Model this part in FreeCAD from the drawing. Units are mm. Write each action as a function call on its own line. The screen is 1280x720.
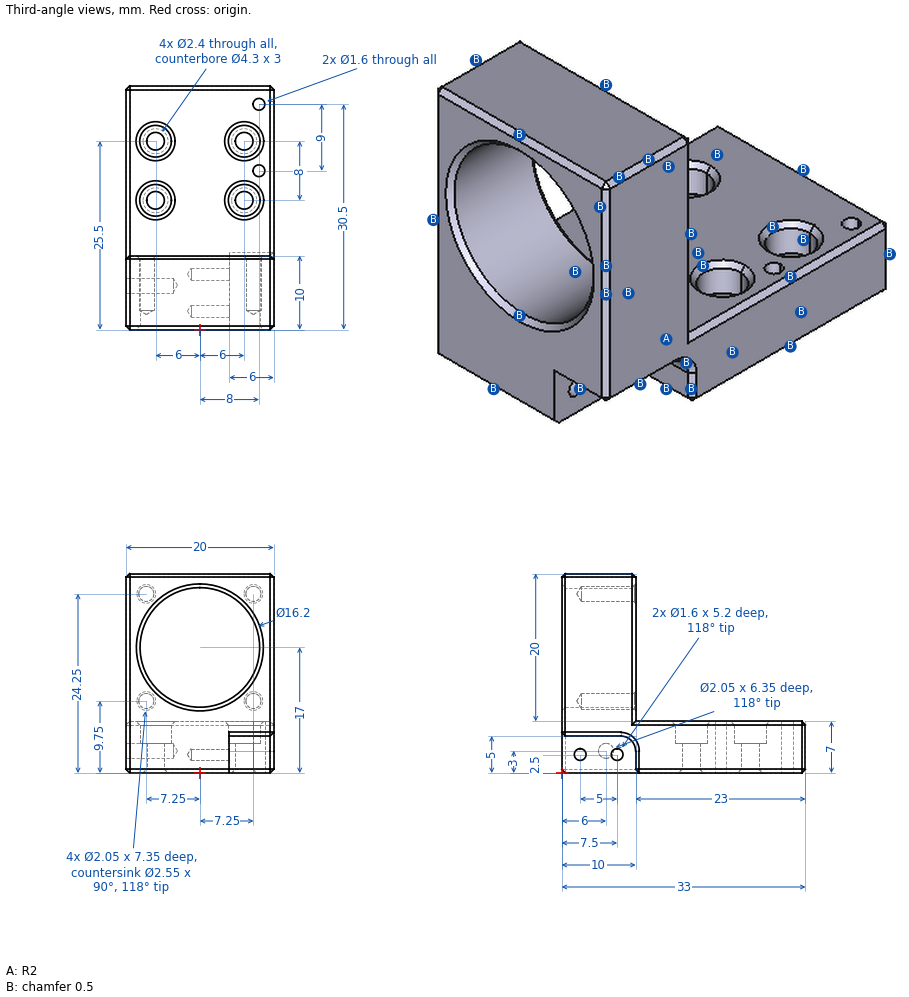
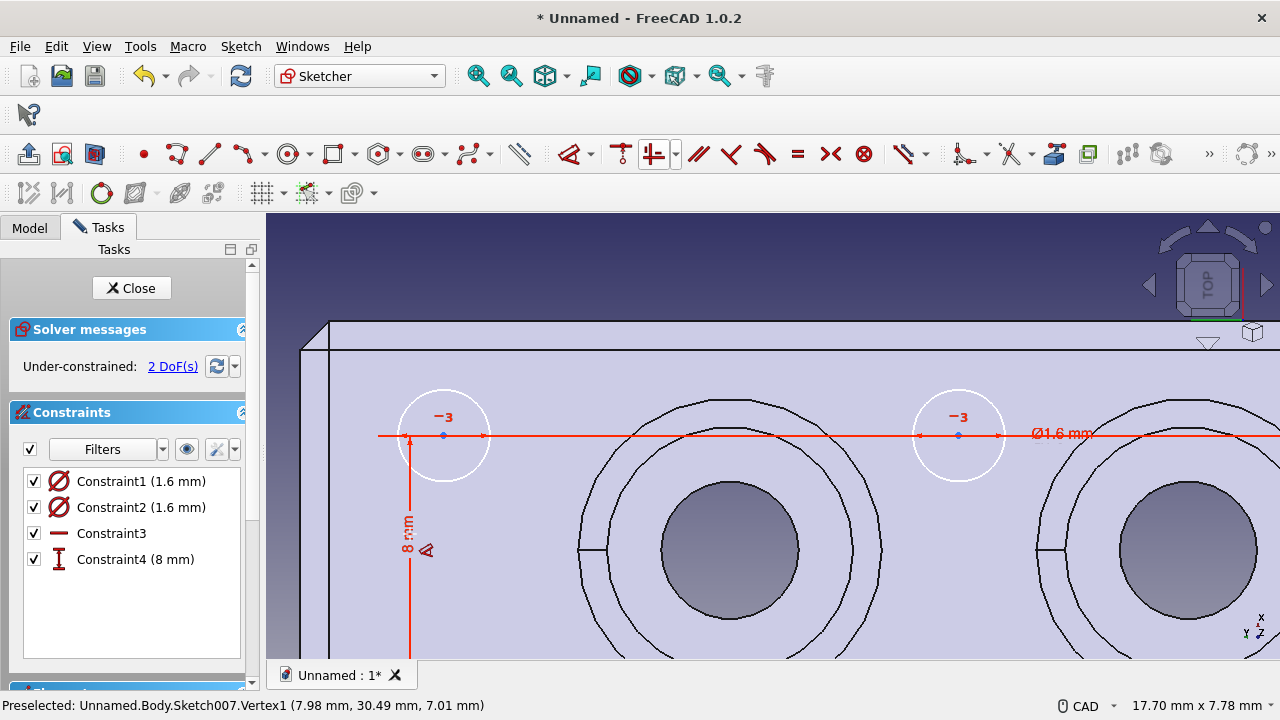
click(444, 436)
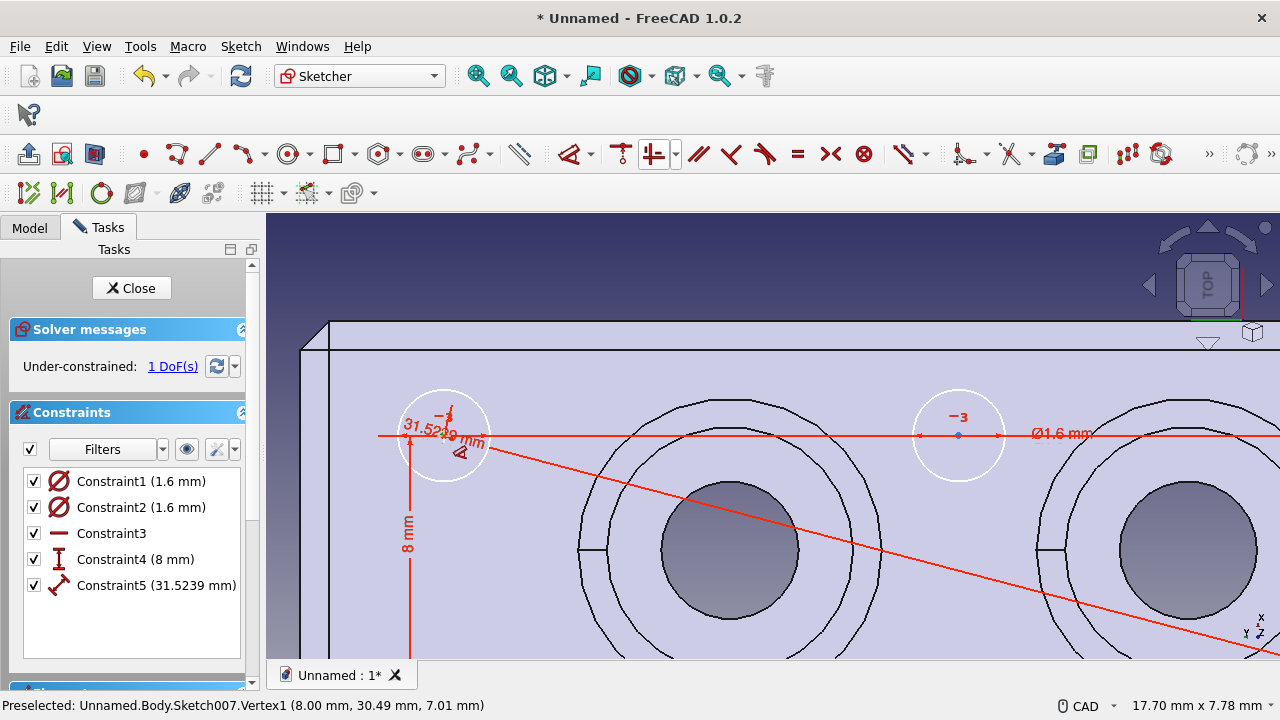
click(959, 436)
click(701, 470)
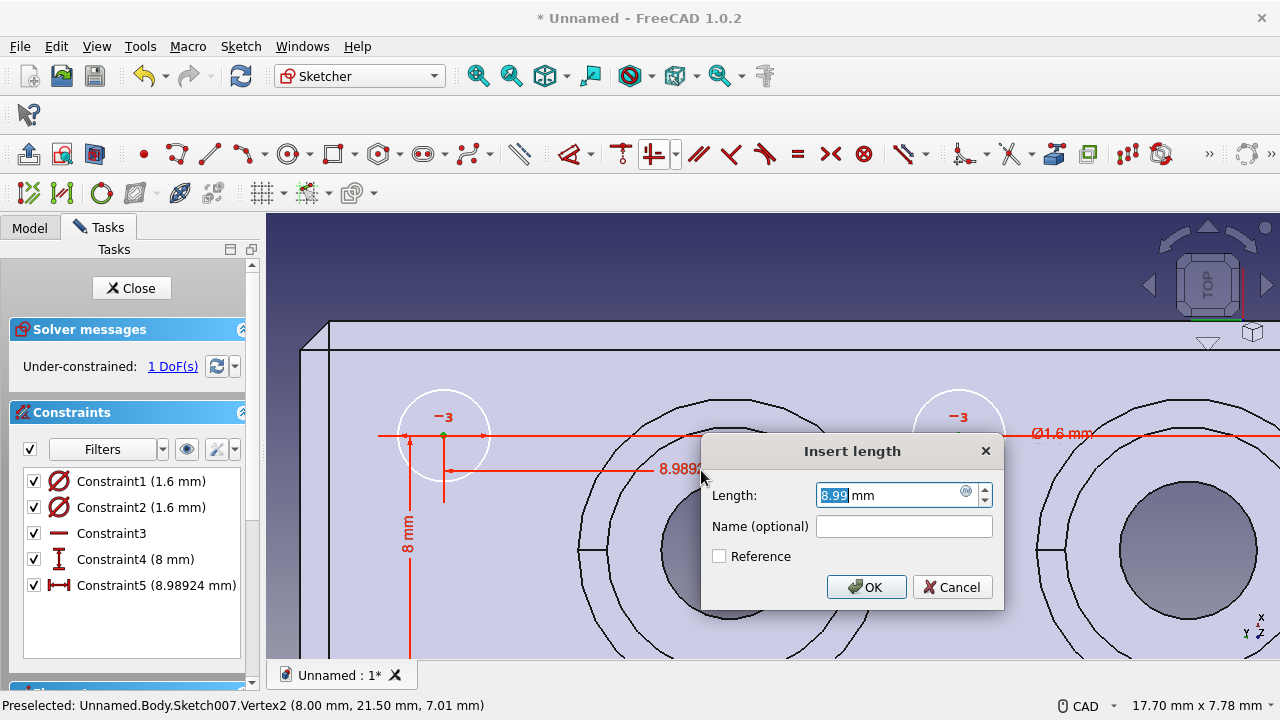
text(9)
key(Return)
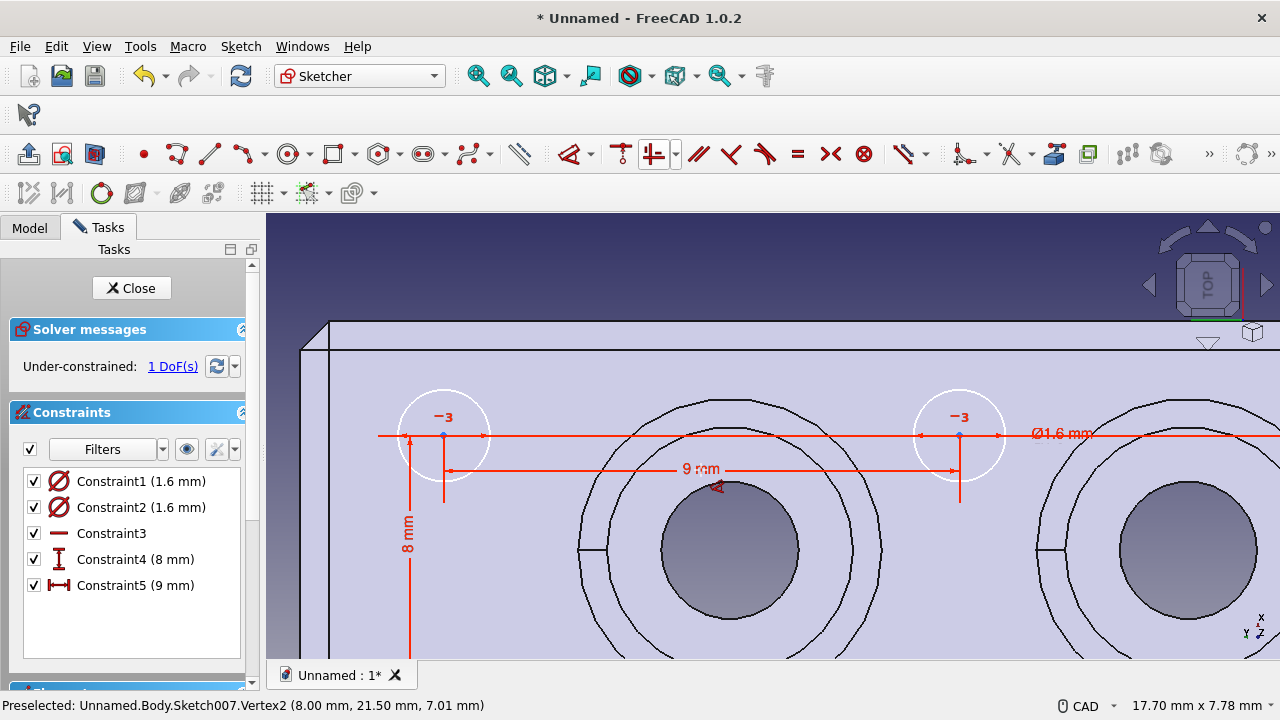
click(444, 436)
click(779, 402)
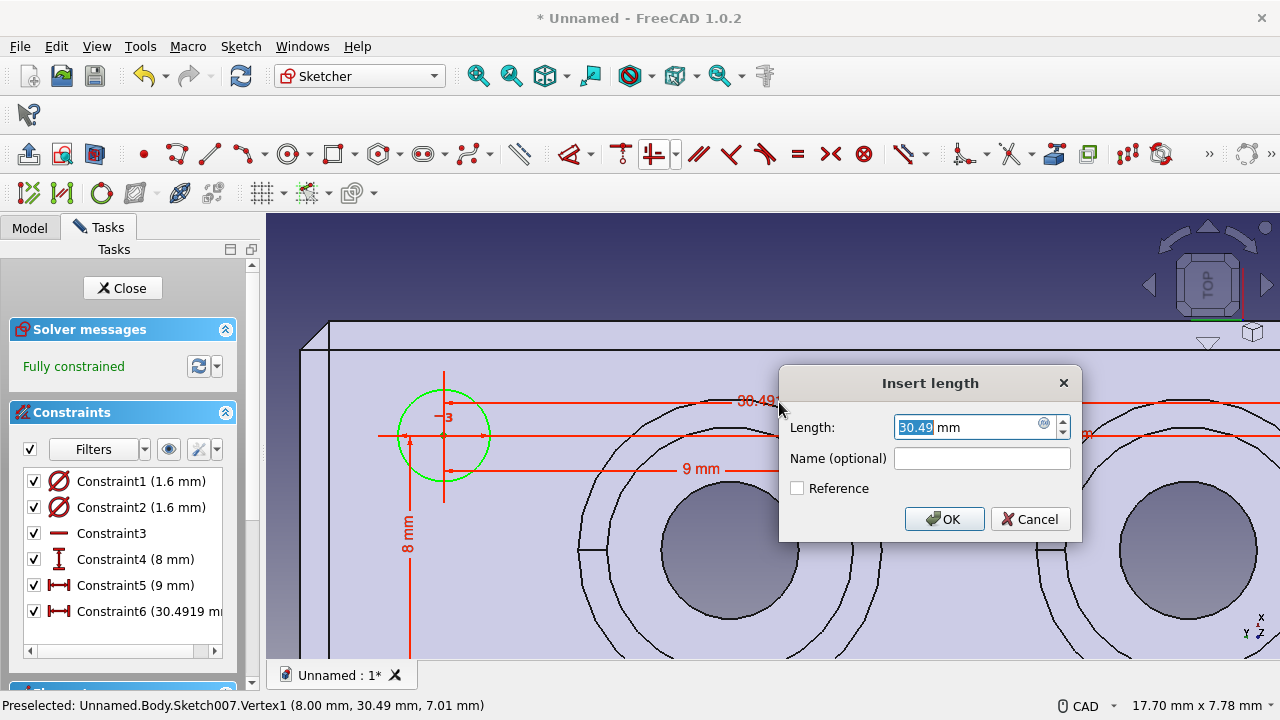
text(30.5)
key(Return)
key(Escape)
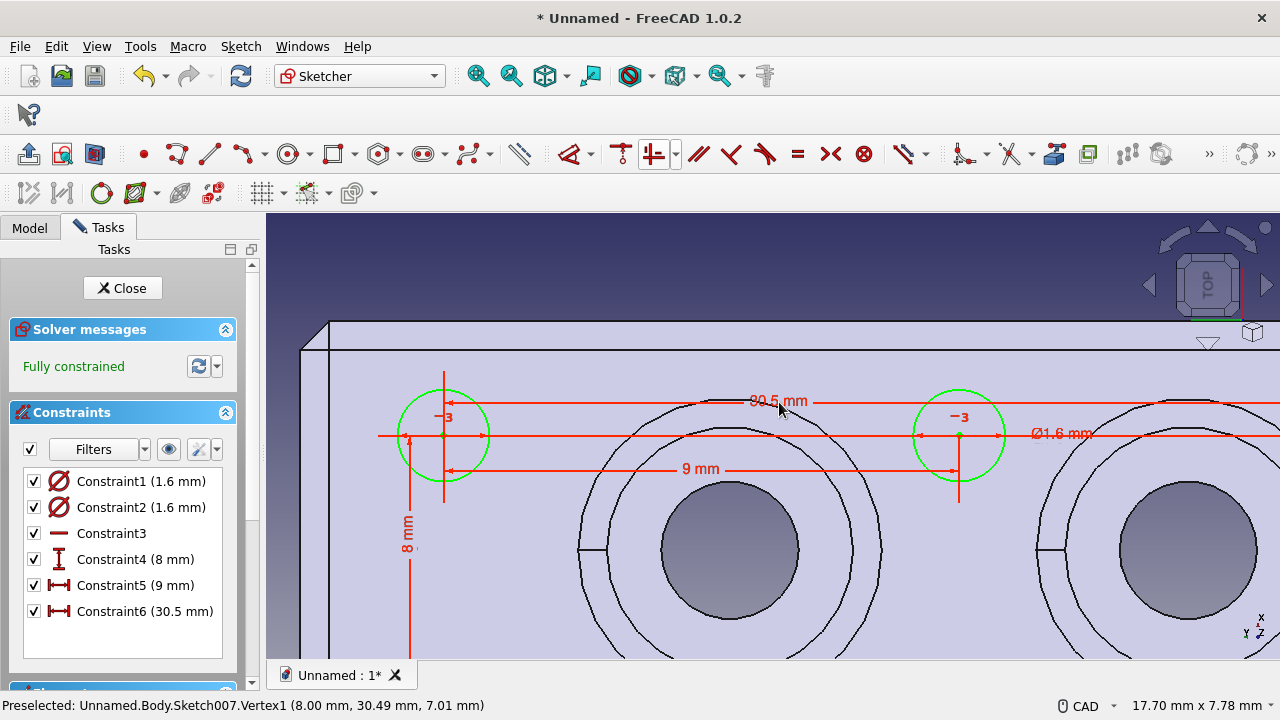
click(123, 288)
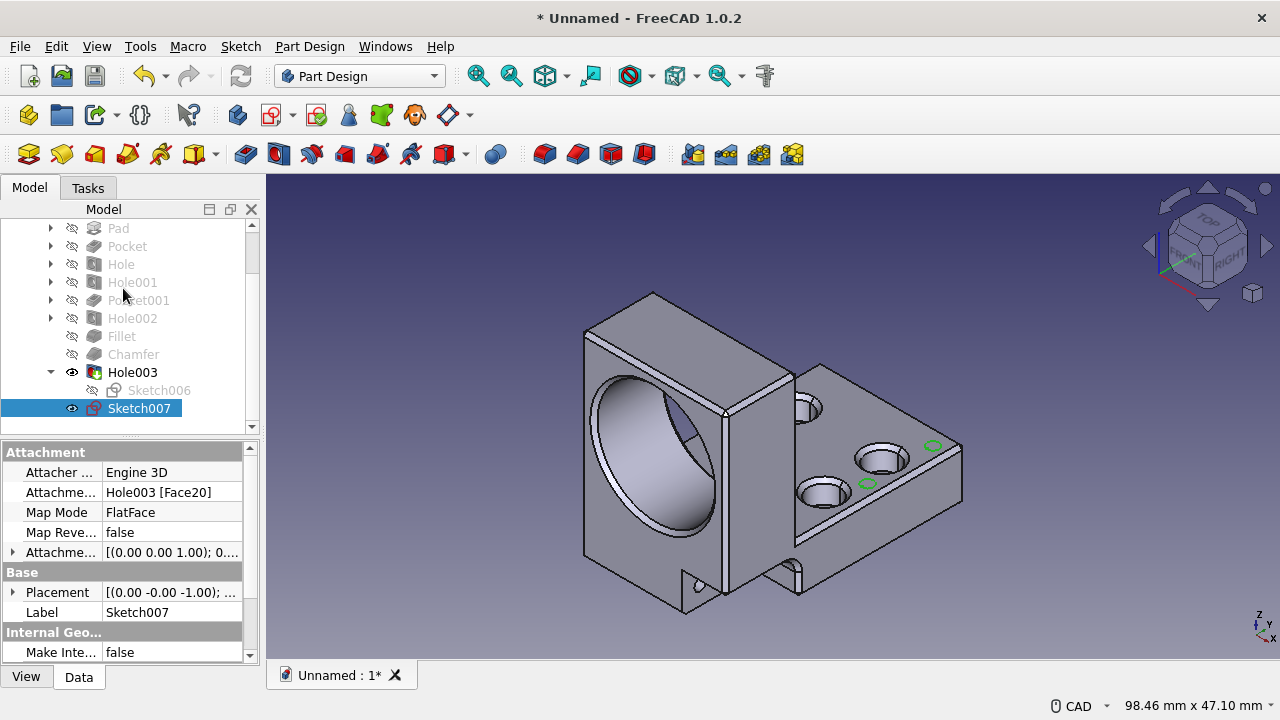
click(279, 154)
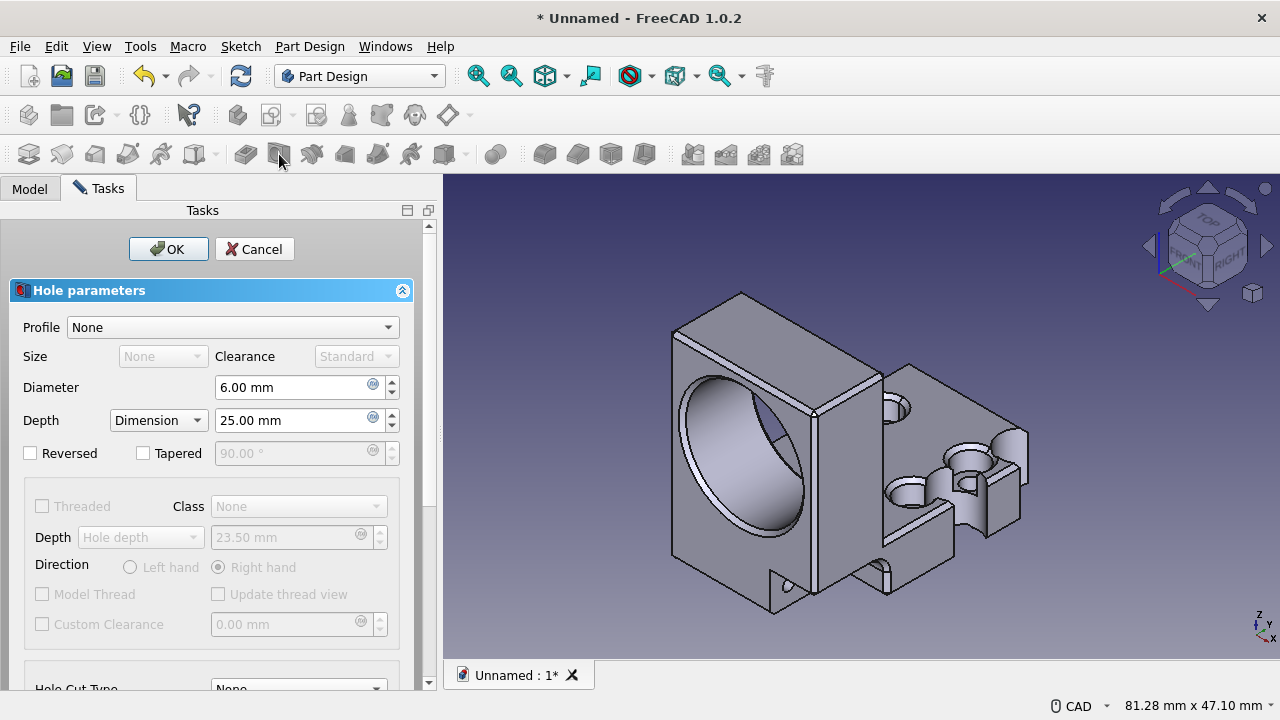
triple_click(300, 388)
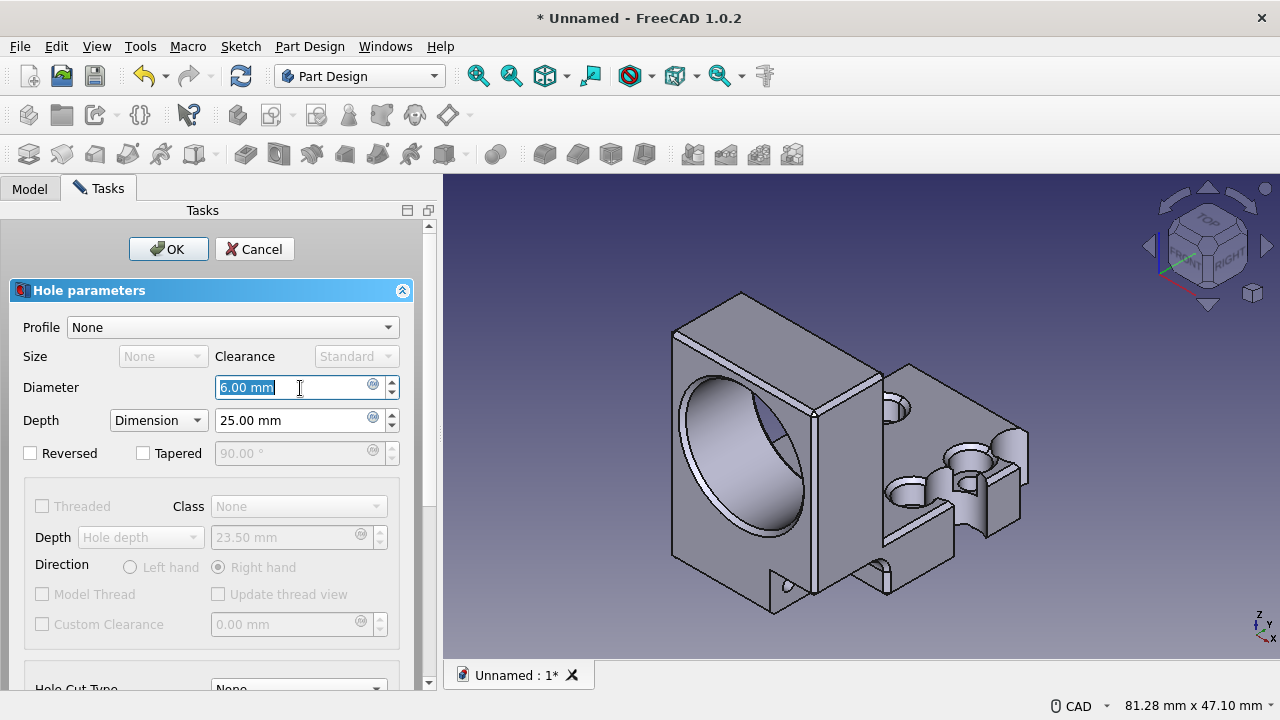
text(1.6)
key(Tab)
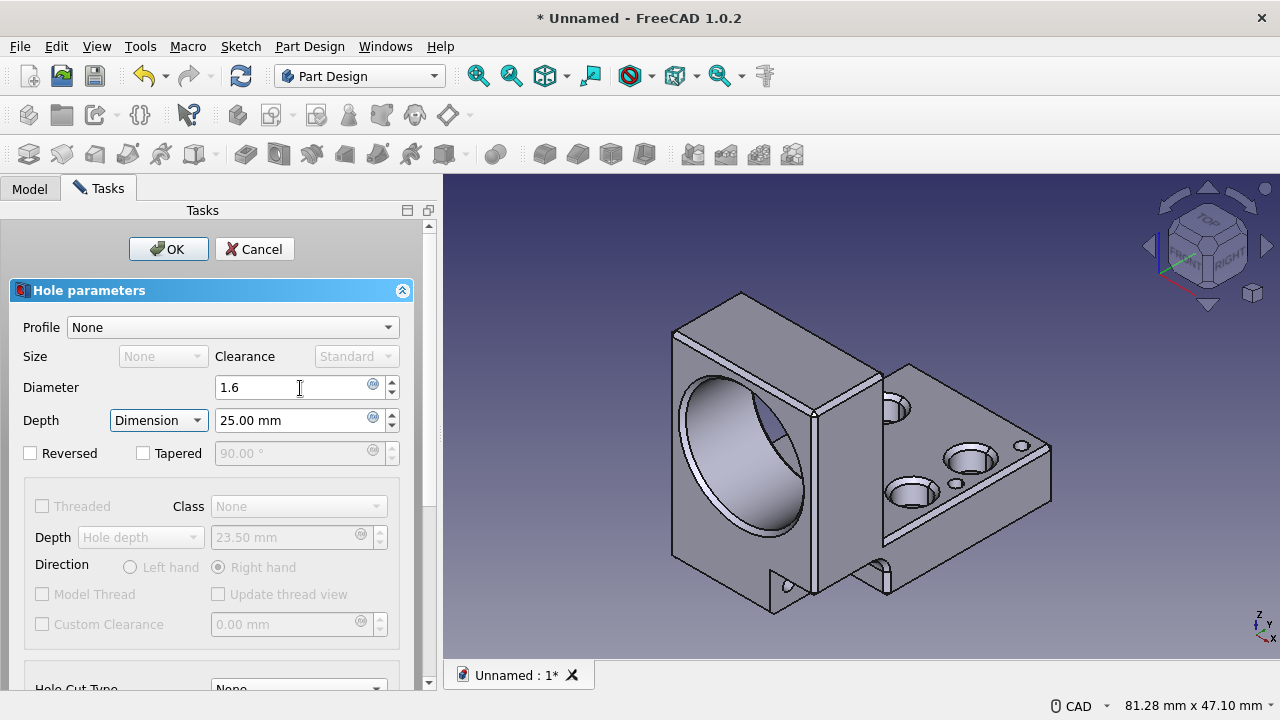
click(160, 420)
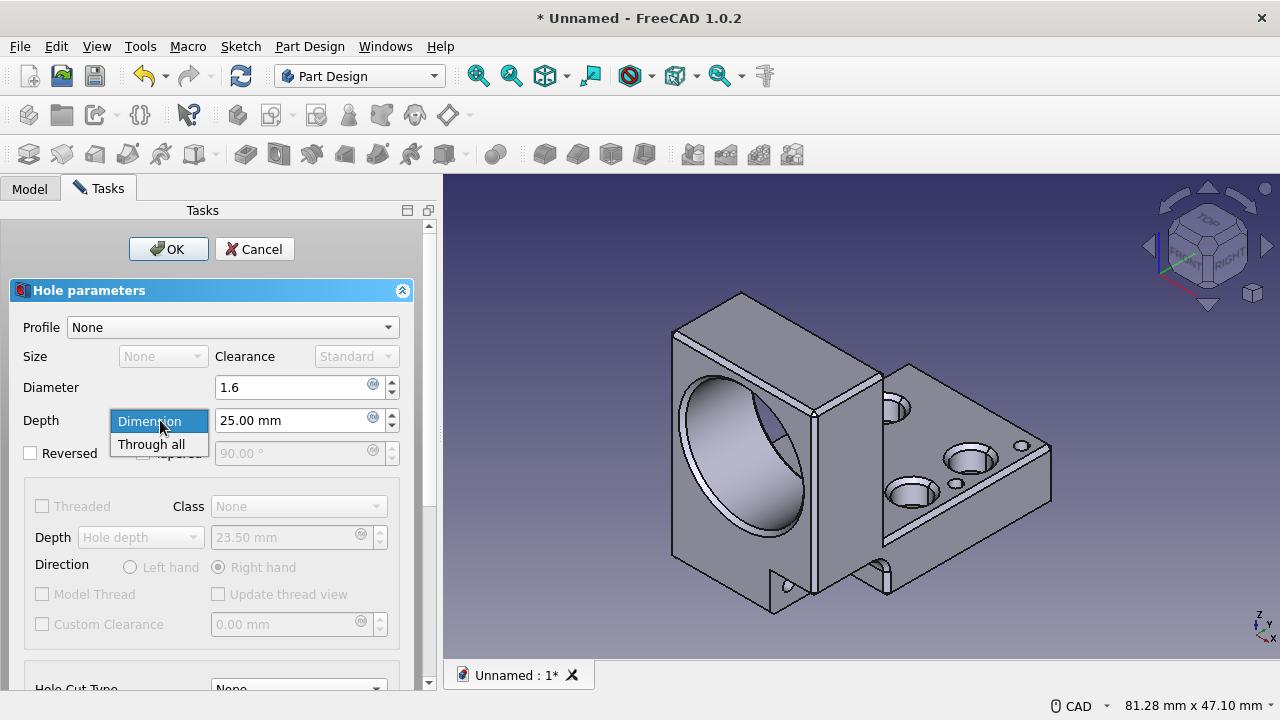
click(158, 444)